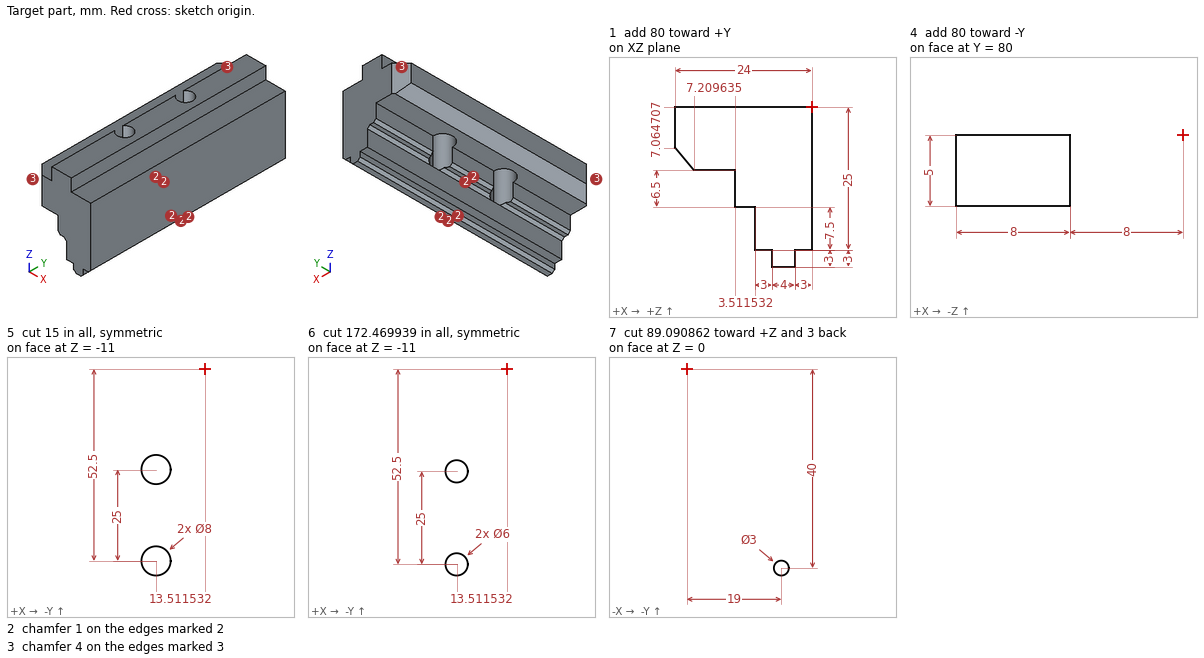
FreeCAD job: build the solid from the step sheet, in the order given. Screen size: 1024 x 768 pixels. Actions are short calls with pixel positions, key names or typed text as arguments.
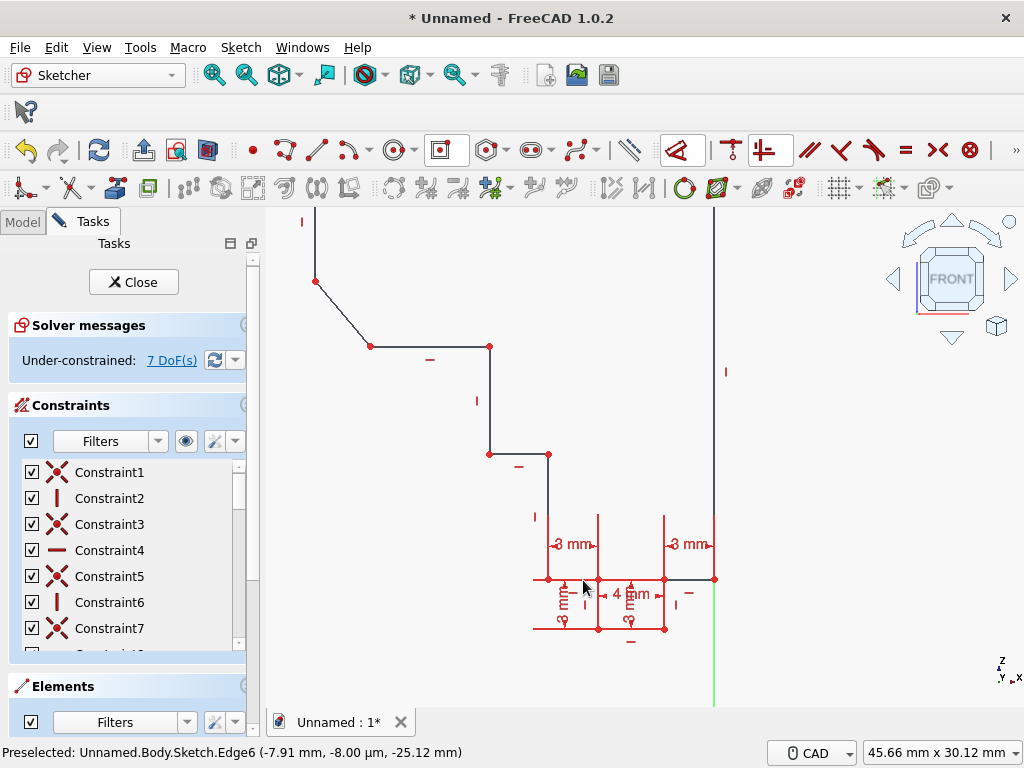
click(714, 288)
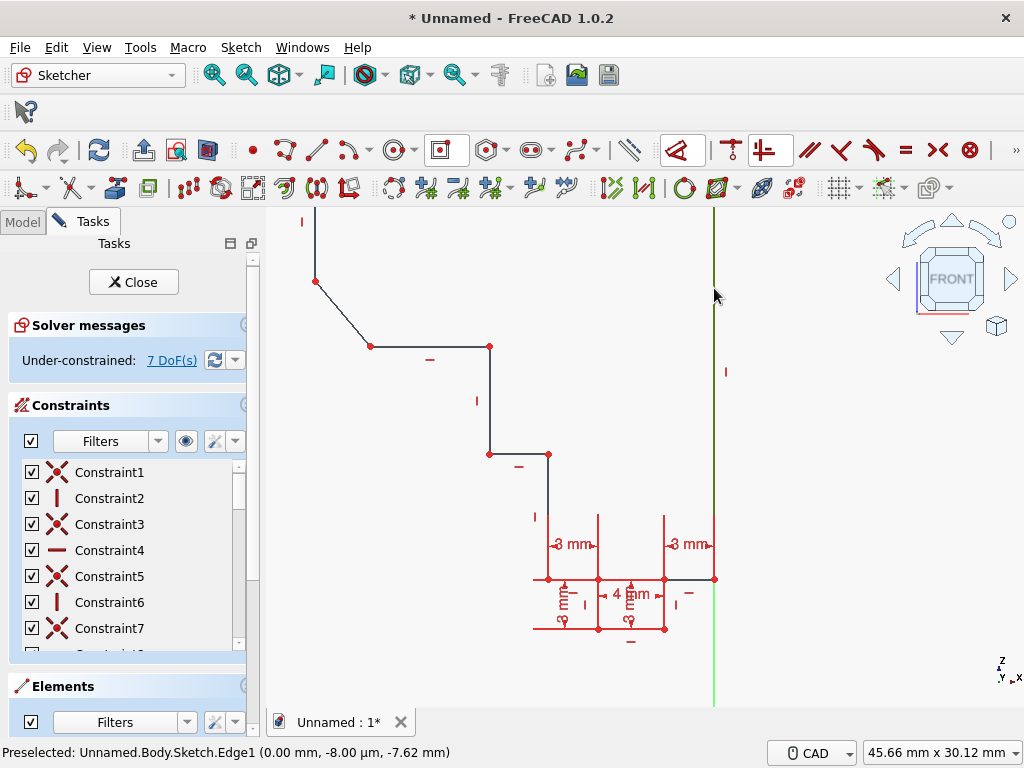
key(i)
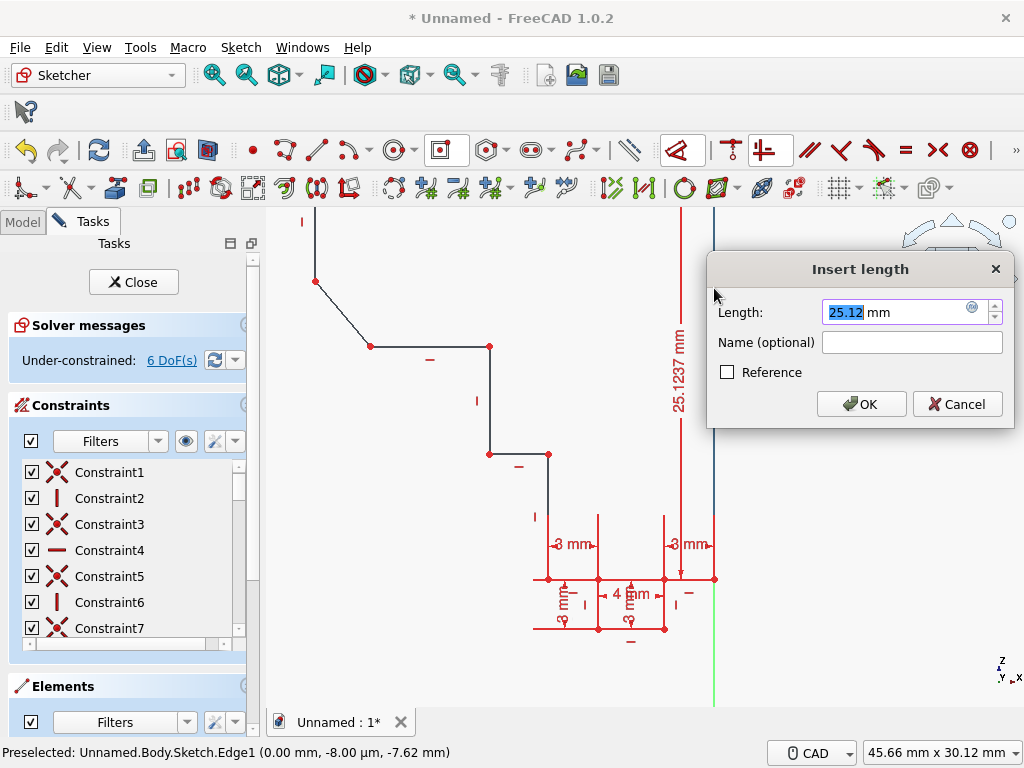
text(25)
key(Return)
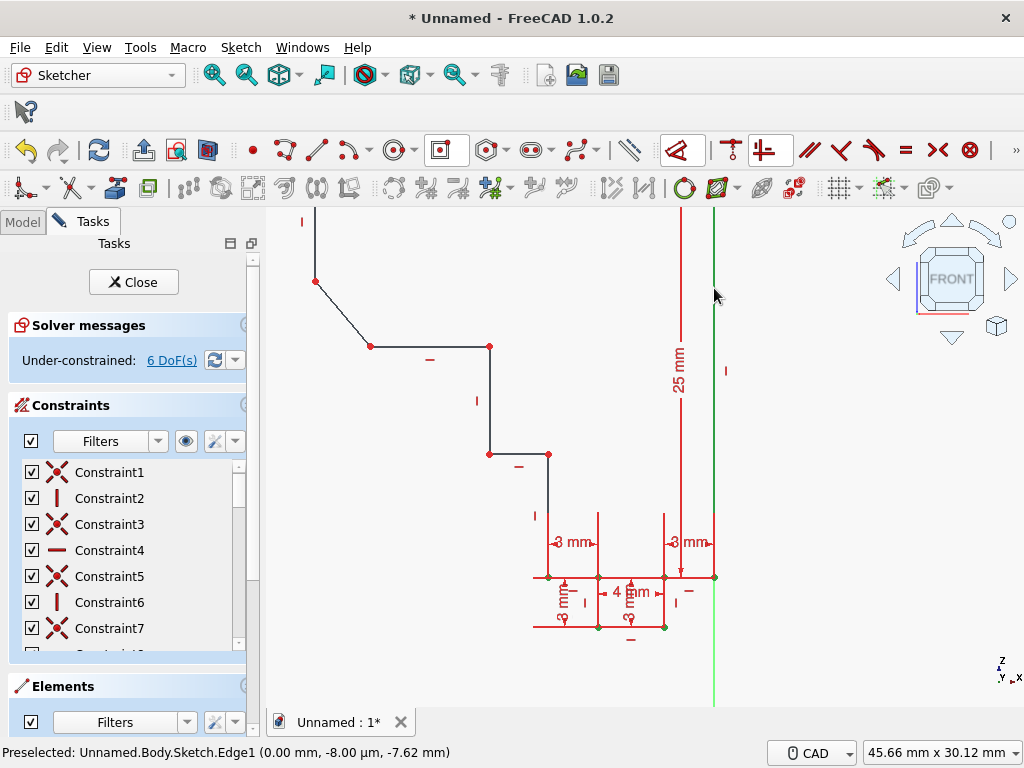
scroll(701, 583, down, 2)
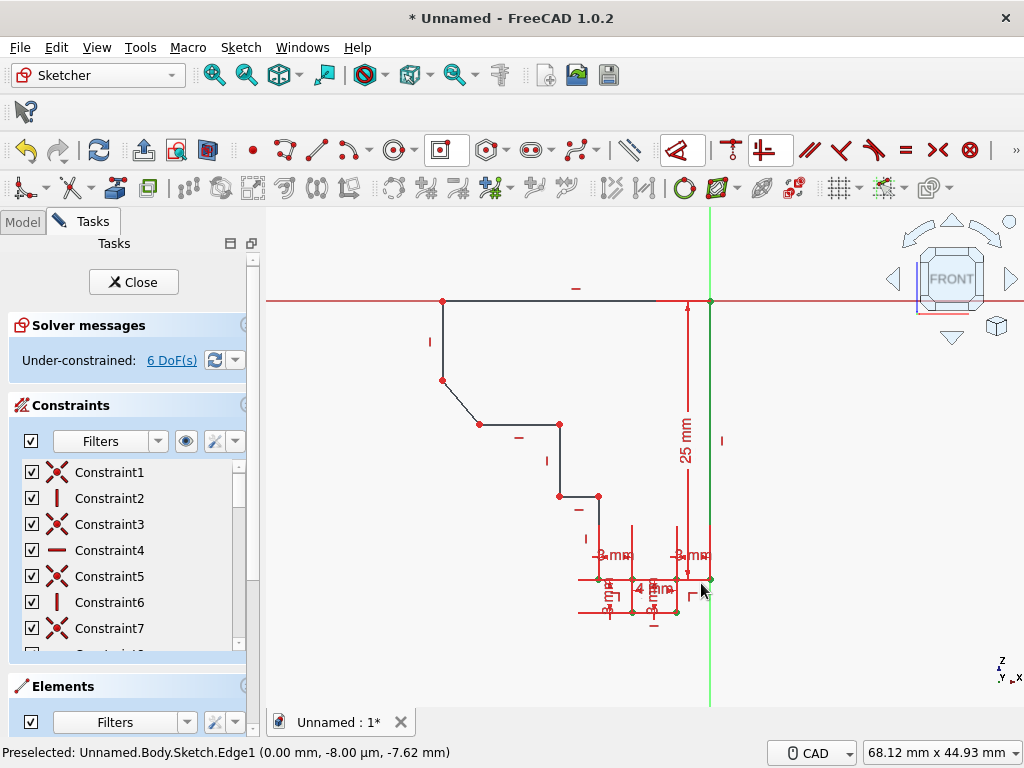
click(523, 301)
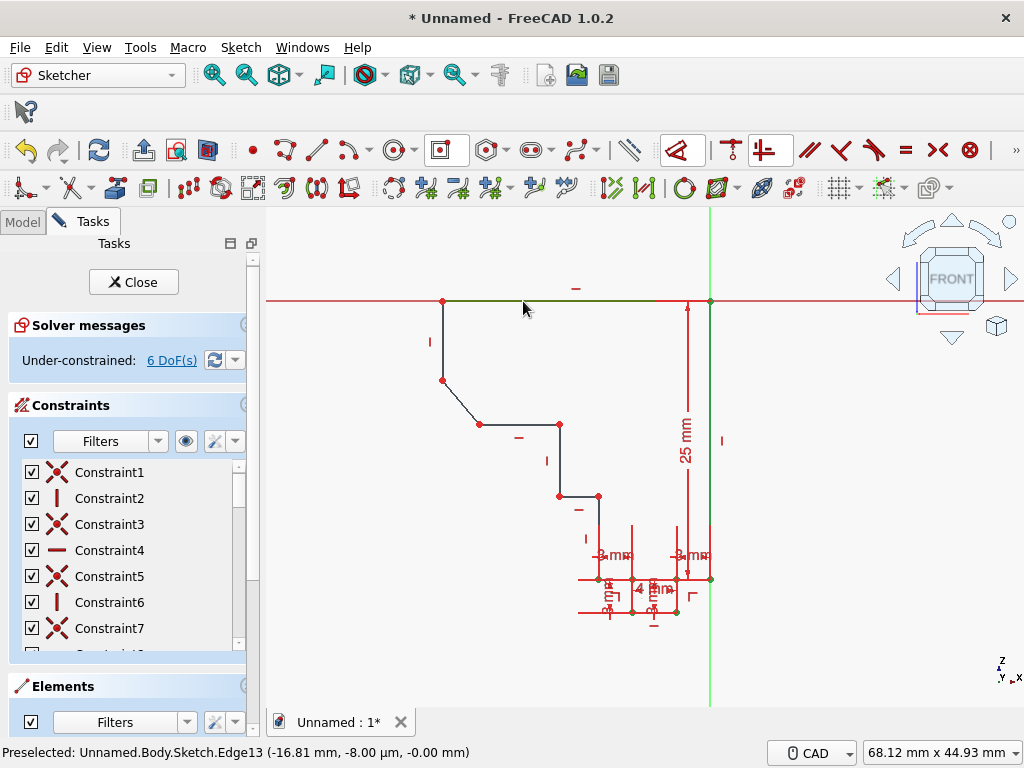
key(l)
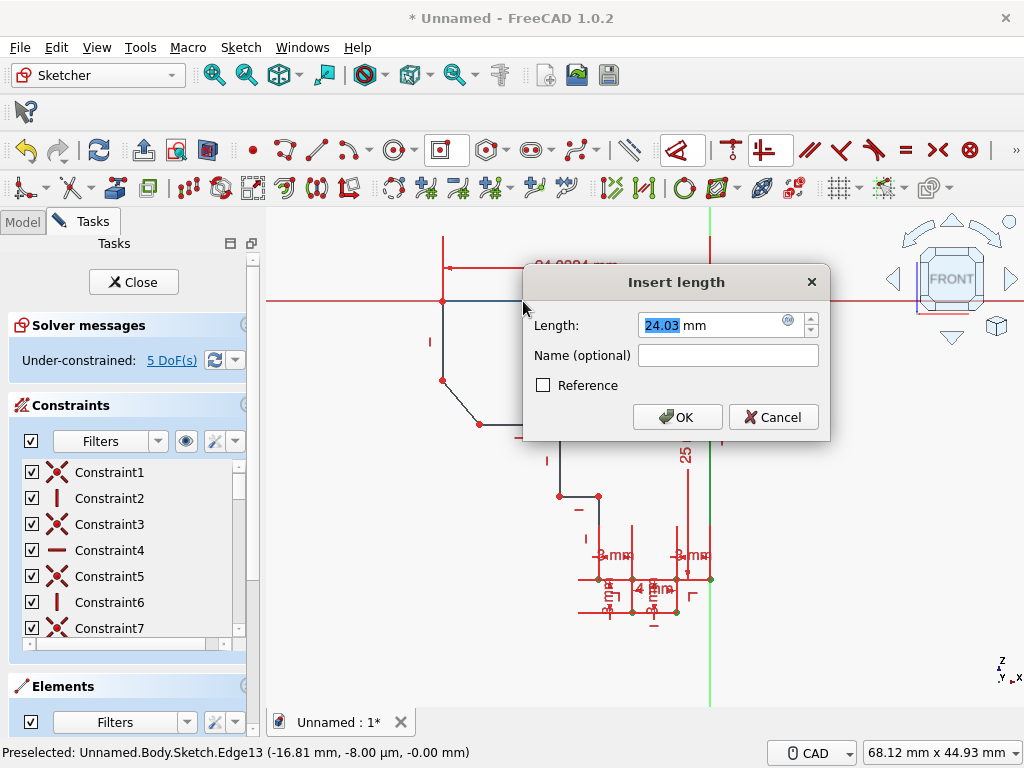
text(24)
key(Return)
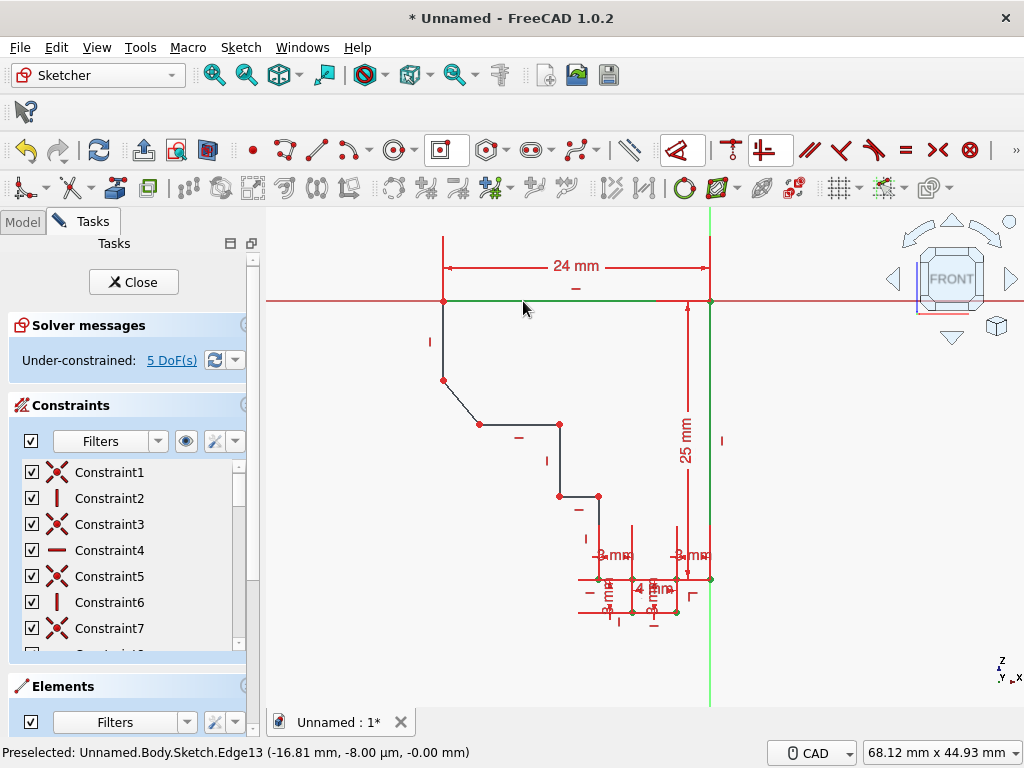
click(599, 522)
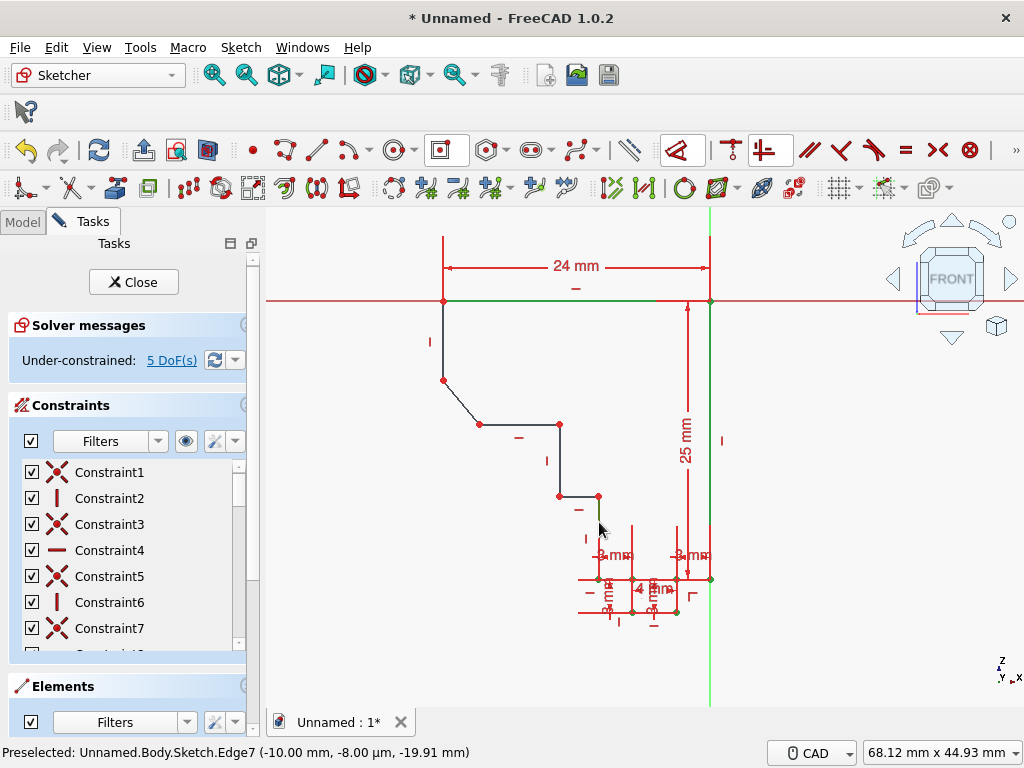
key(i)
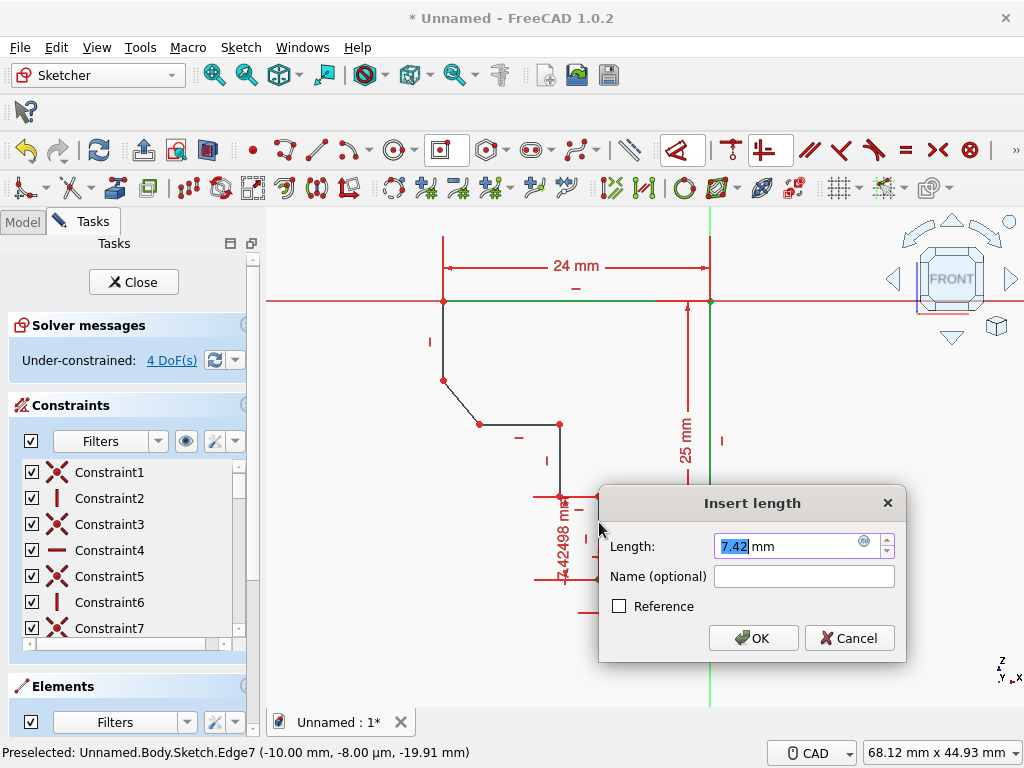
text(7.5)
key(Return)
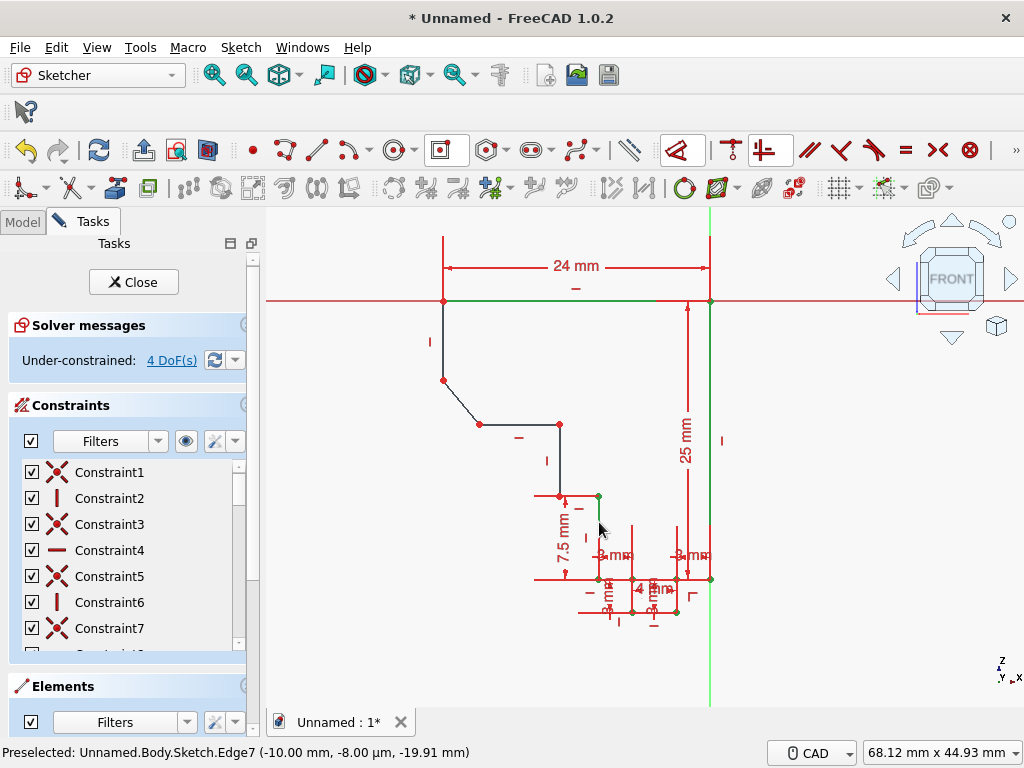
click(560, 475)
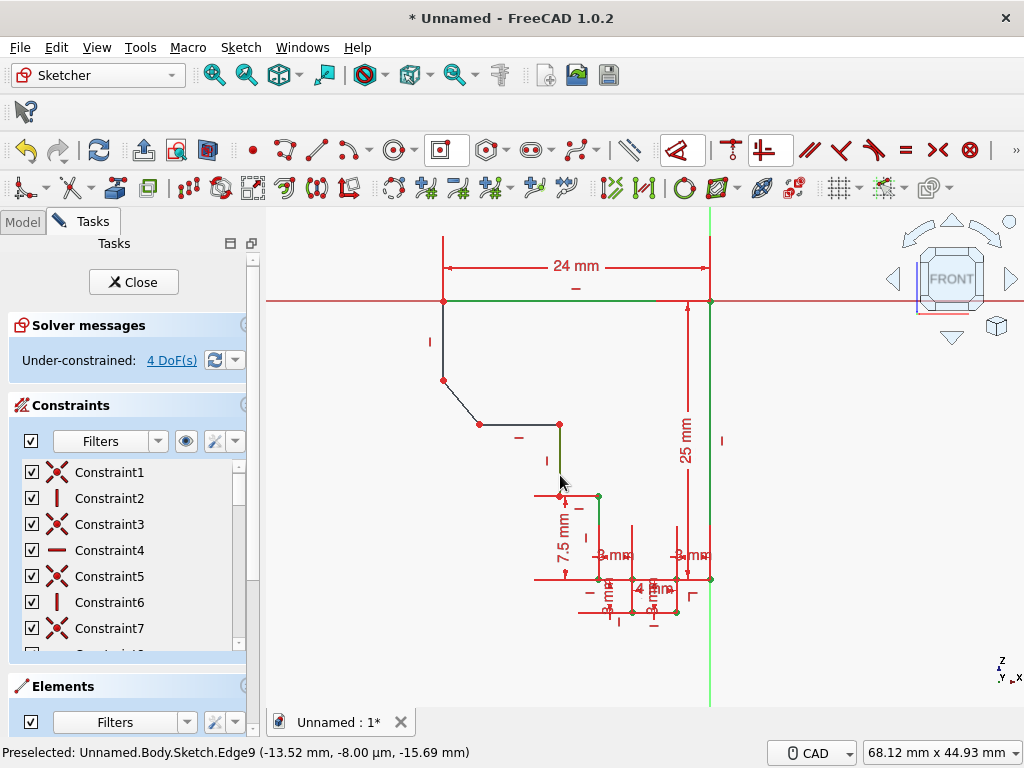
key(i)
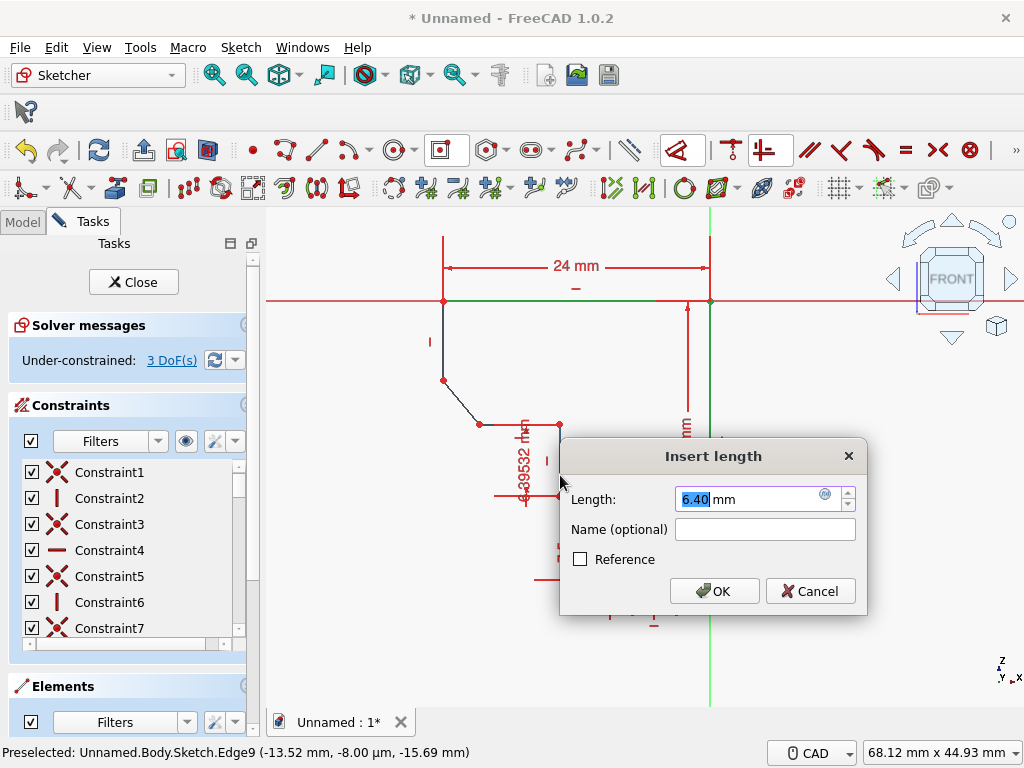
text(6.5)
key(Return)